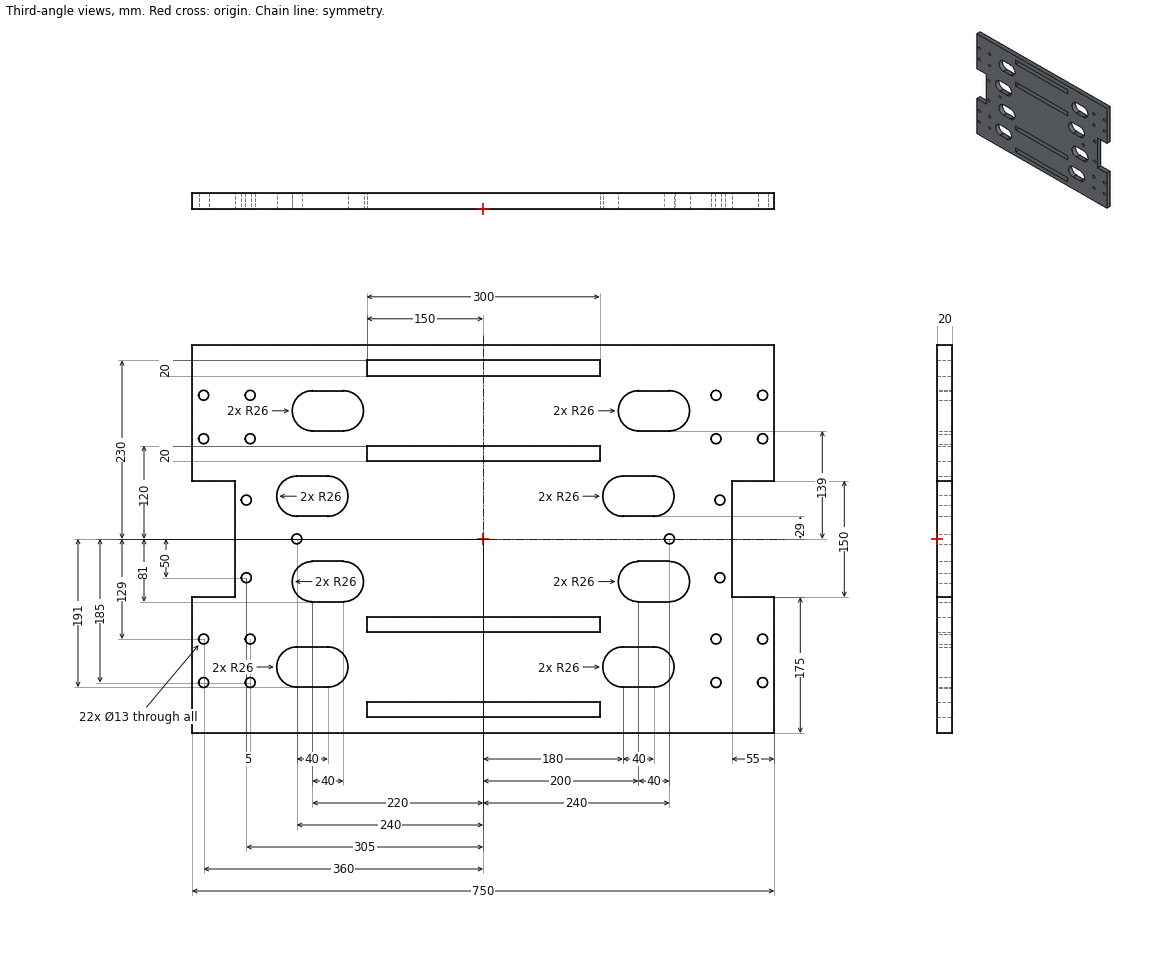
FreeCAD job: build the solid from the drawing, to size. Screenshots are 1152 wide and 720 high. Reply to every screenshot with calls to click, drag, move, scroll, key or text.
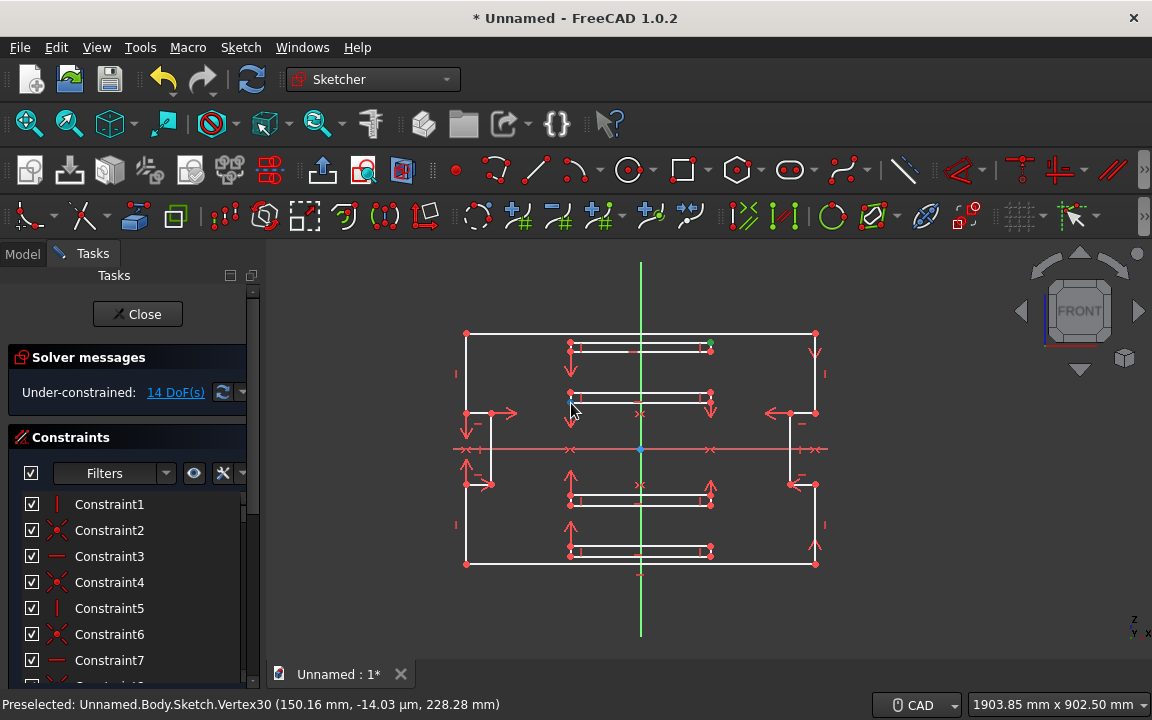
click(711, 557)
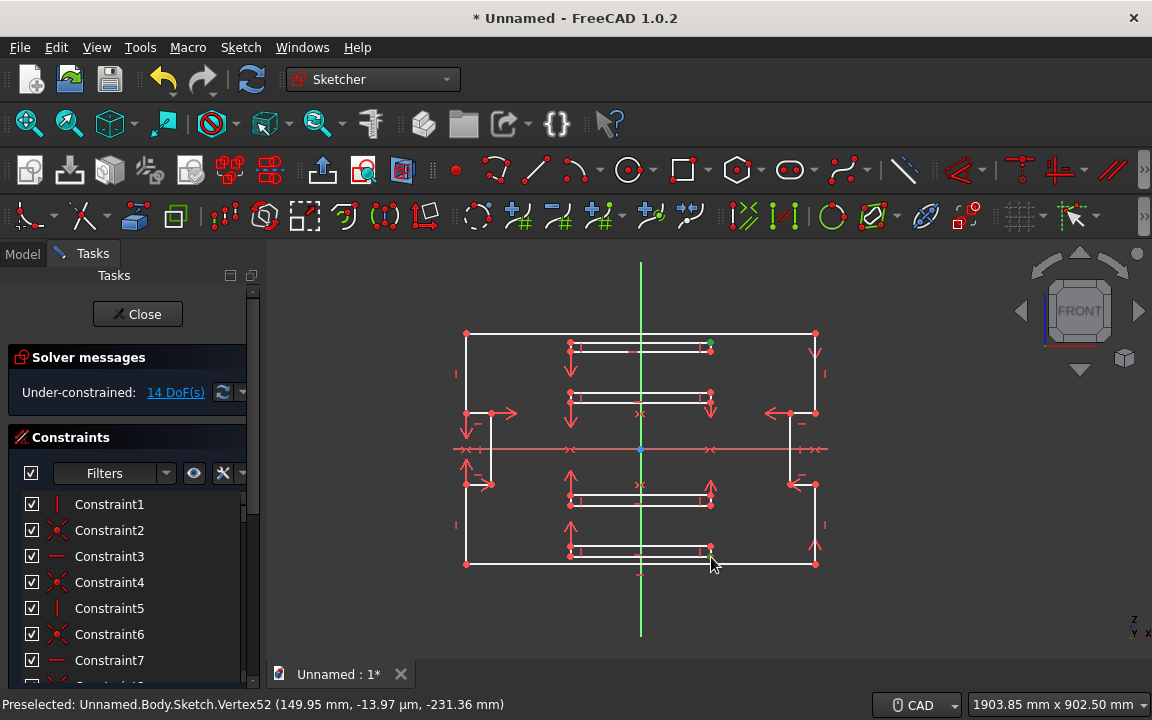
click(542, 449)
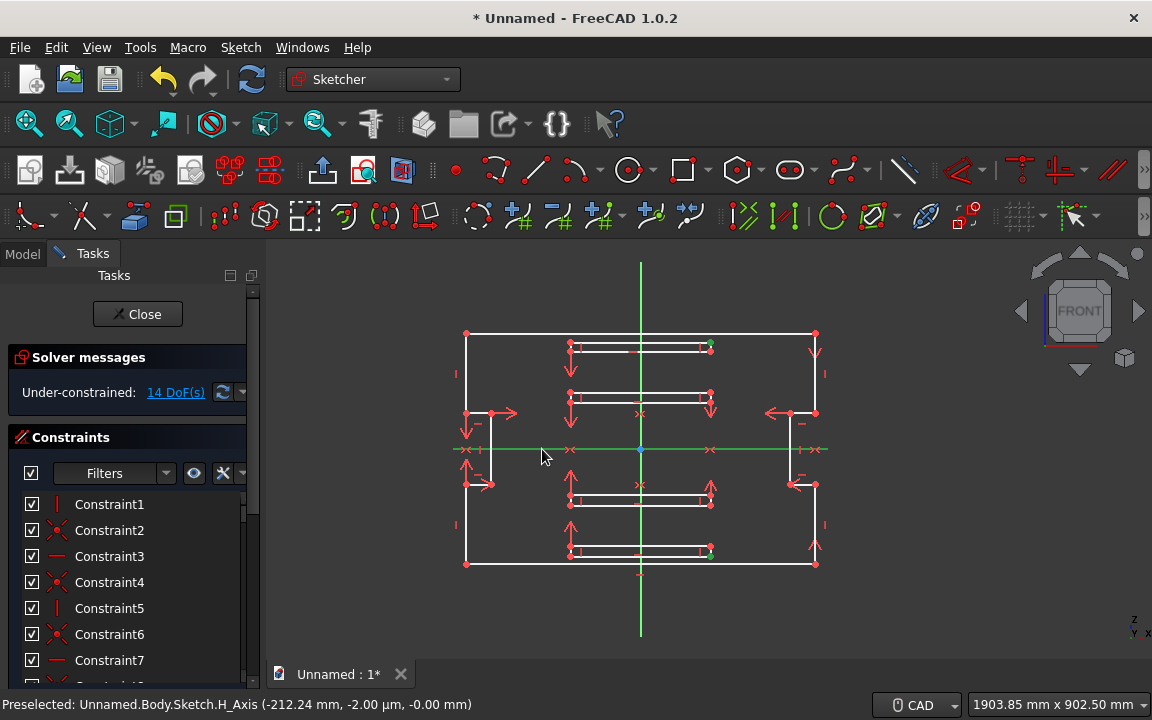
key(s)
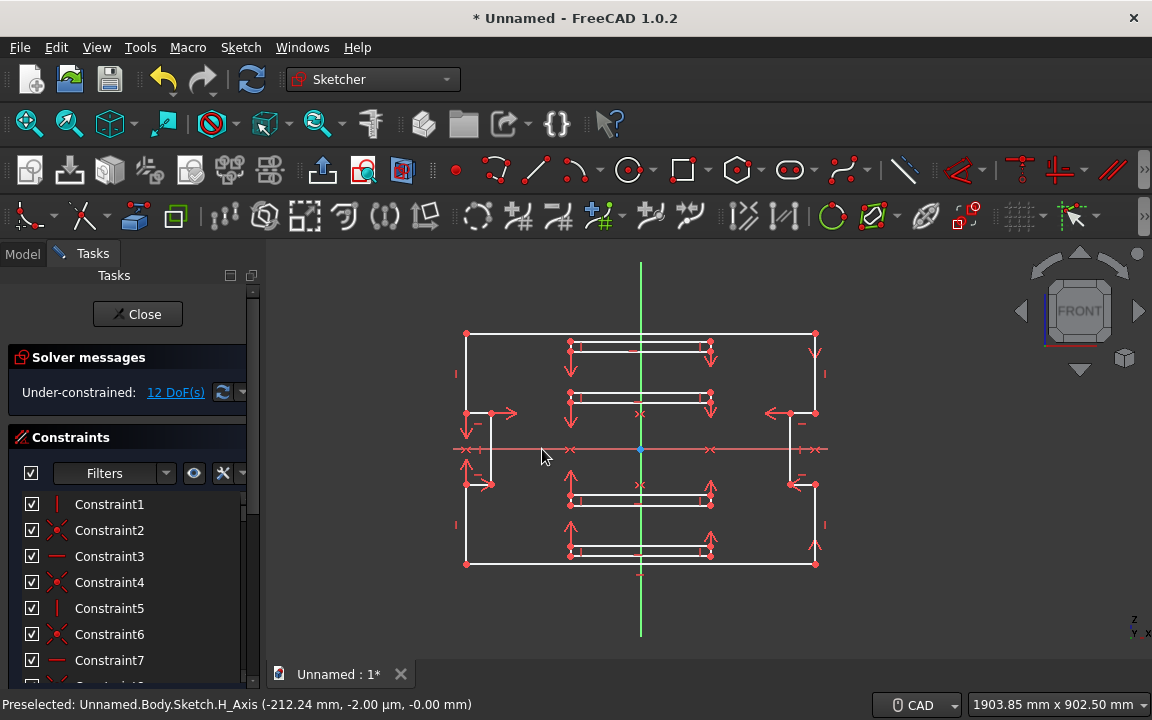
click(958, 170)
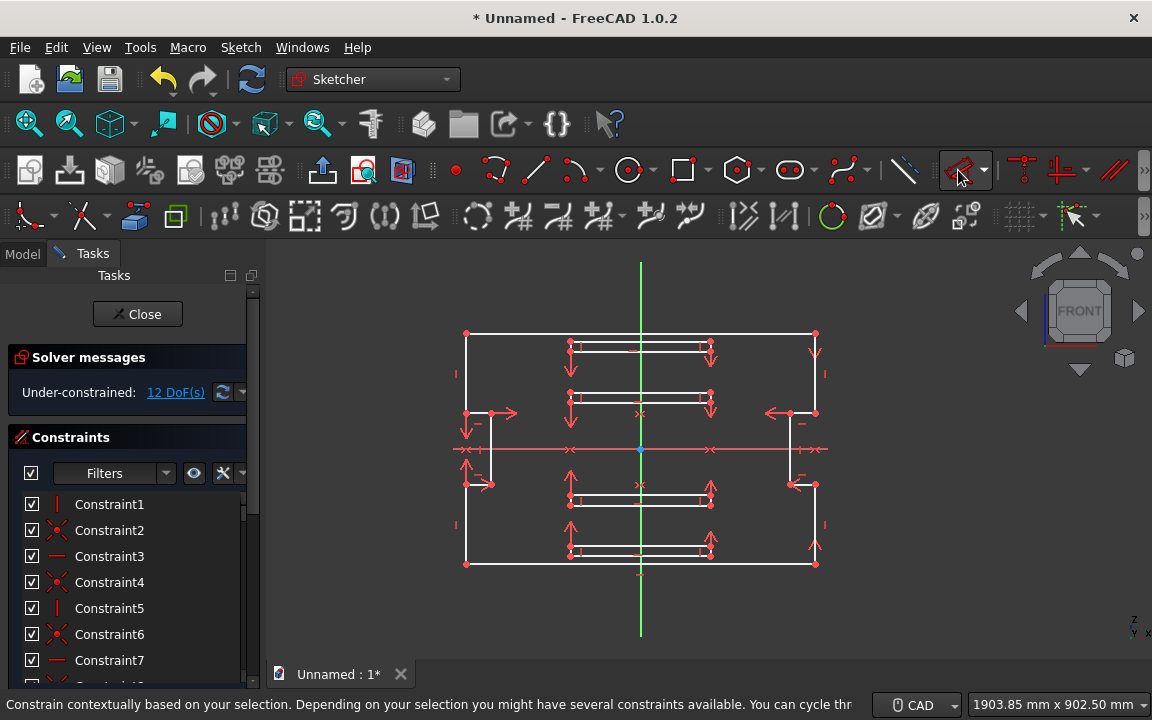
scroll(800, 485, up, 3)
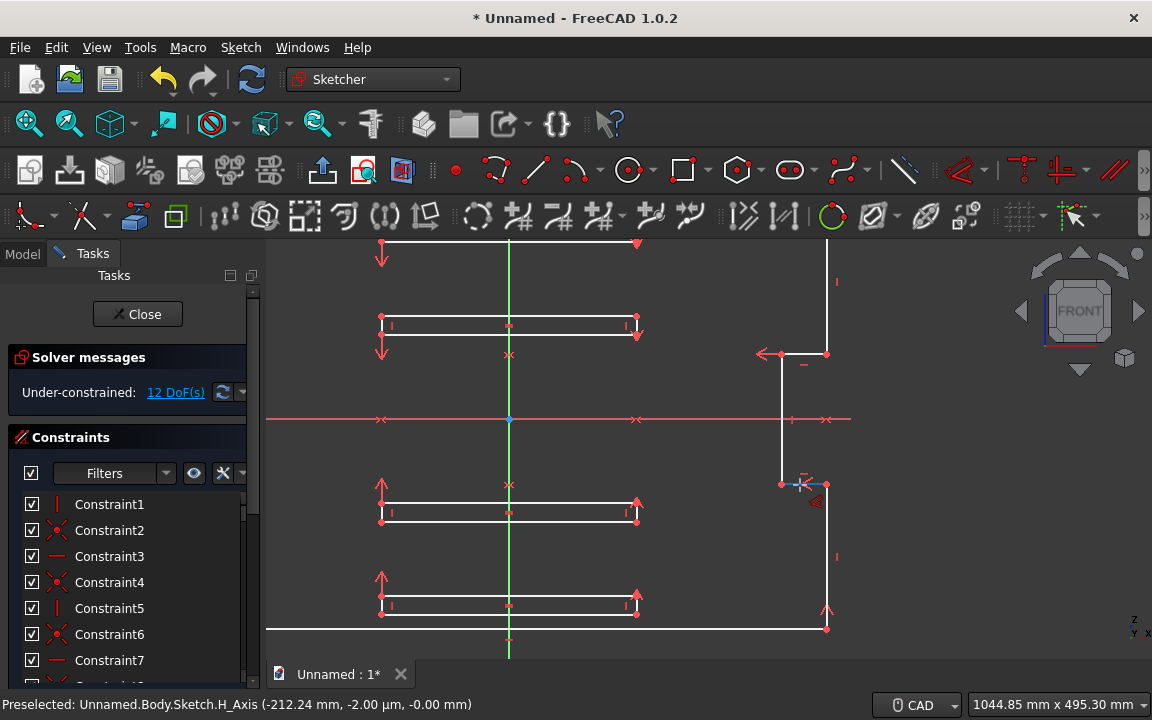
click(800, 484)
click(804, 518)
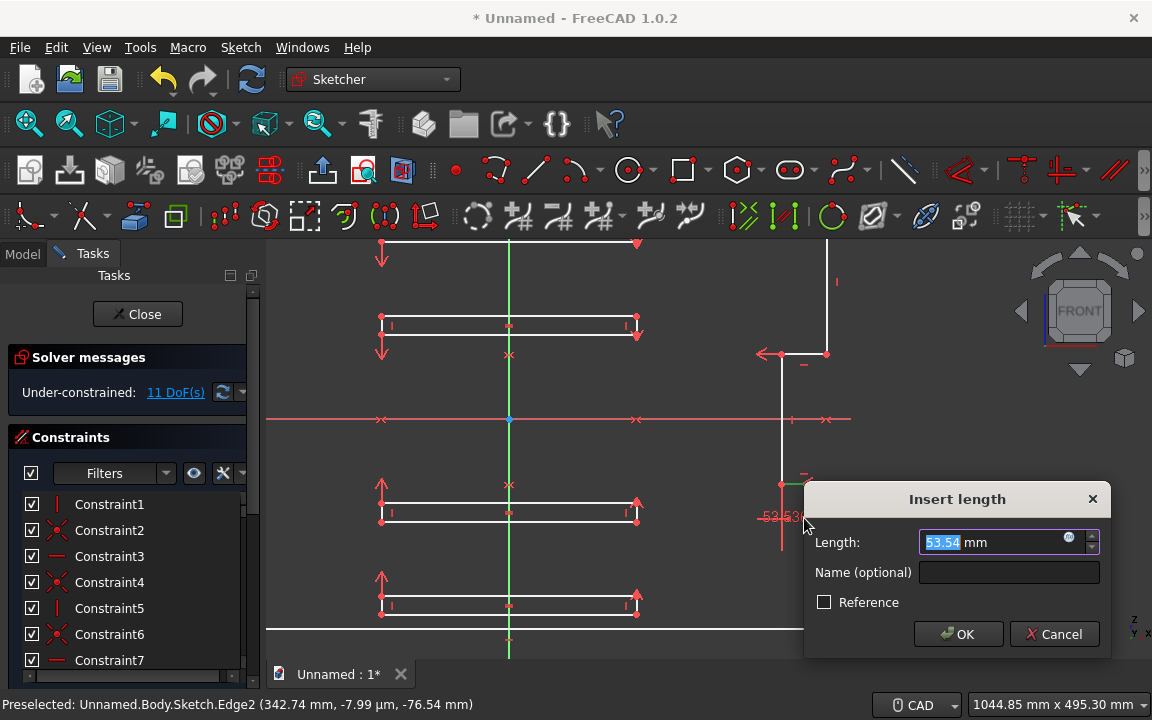
text(55)
key(Return)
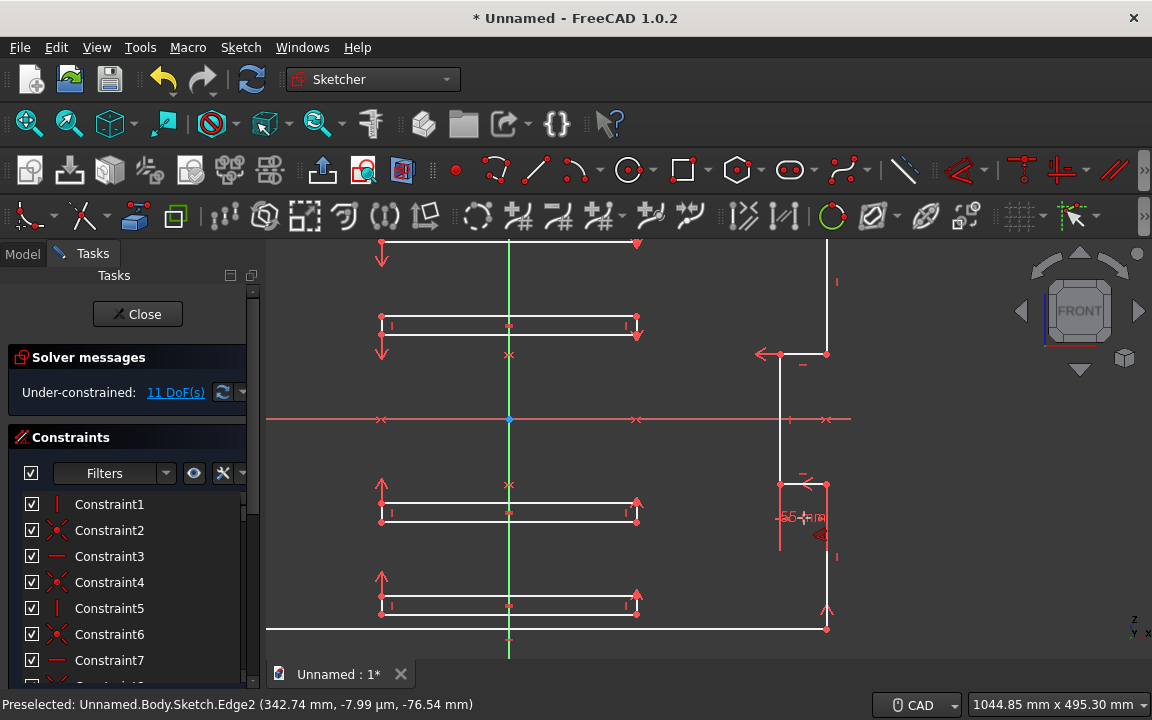
scroll(800, 485, down, 3)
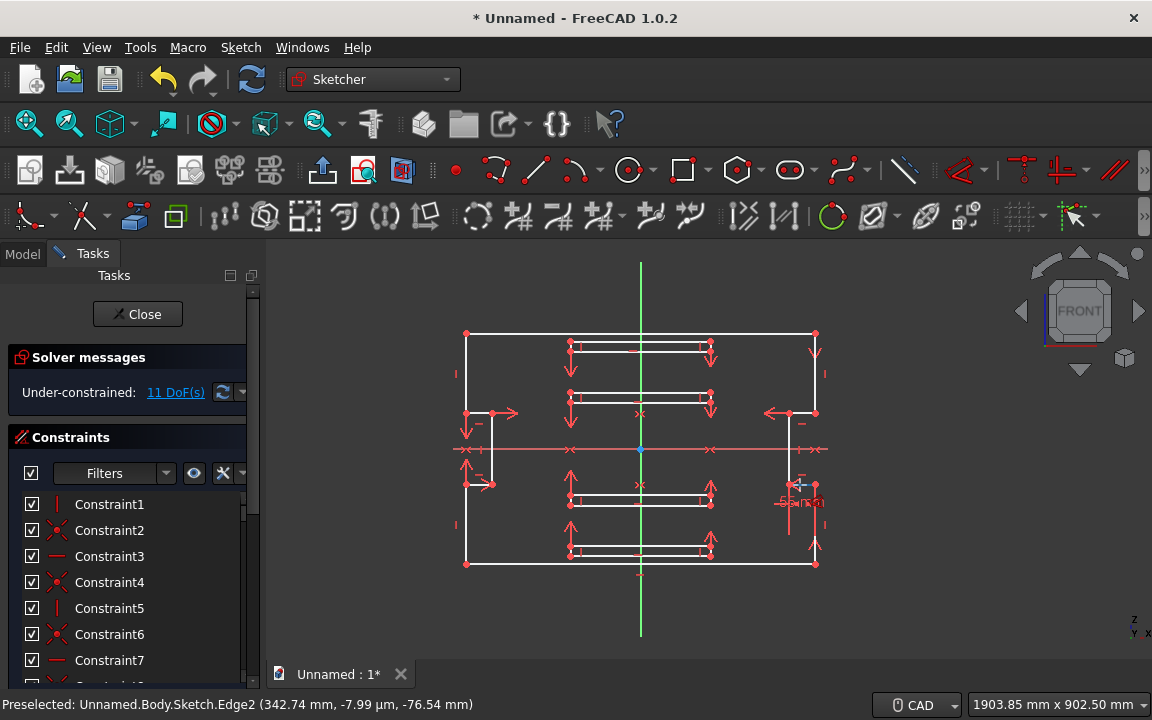
scroll(571, 347, up, 8)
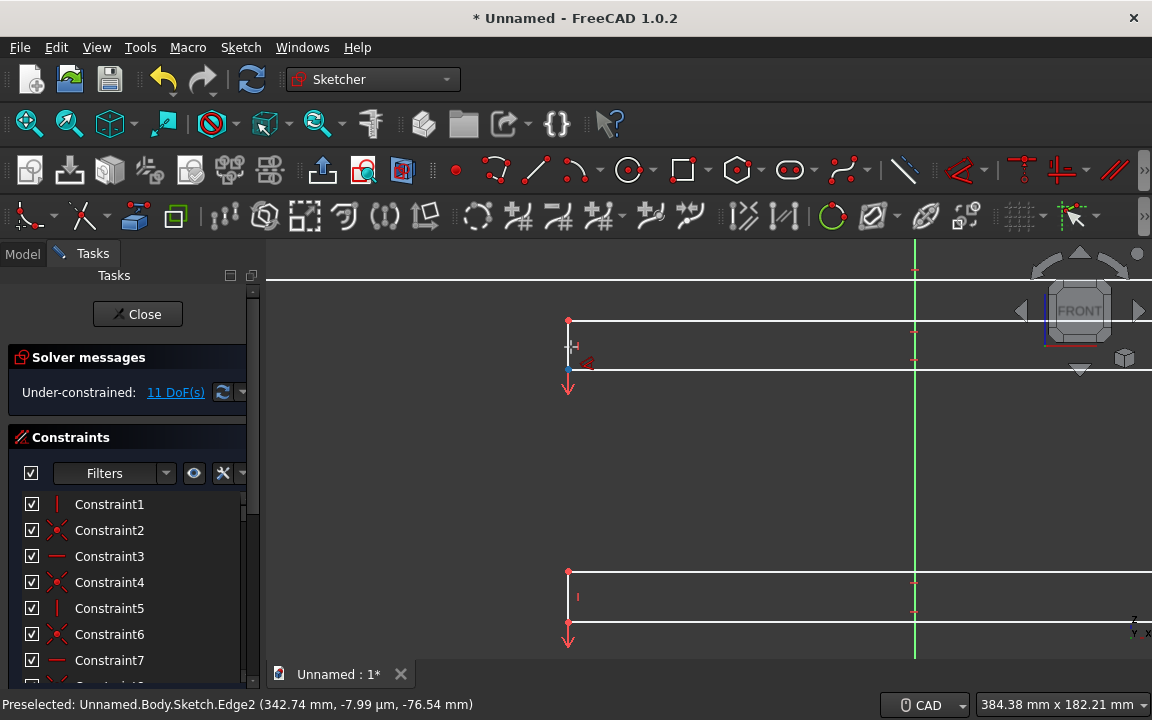
click(568, 345)
click(534, 345)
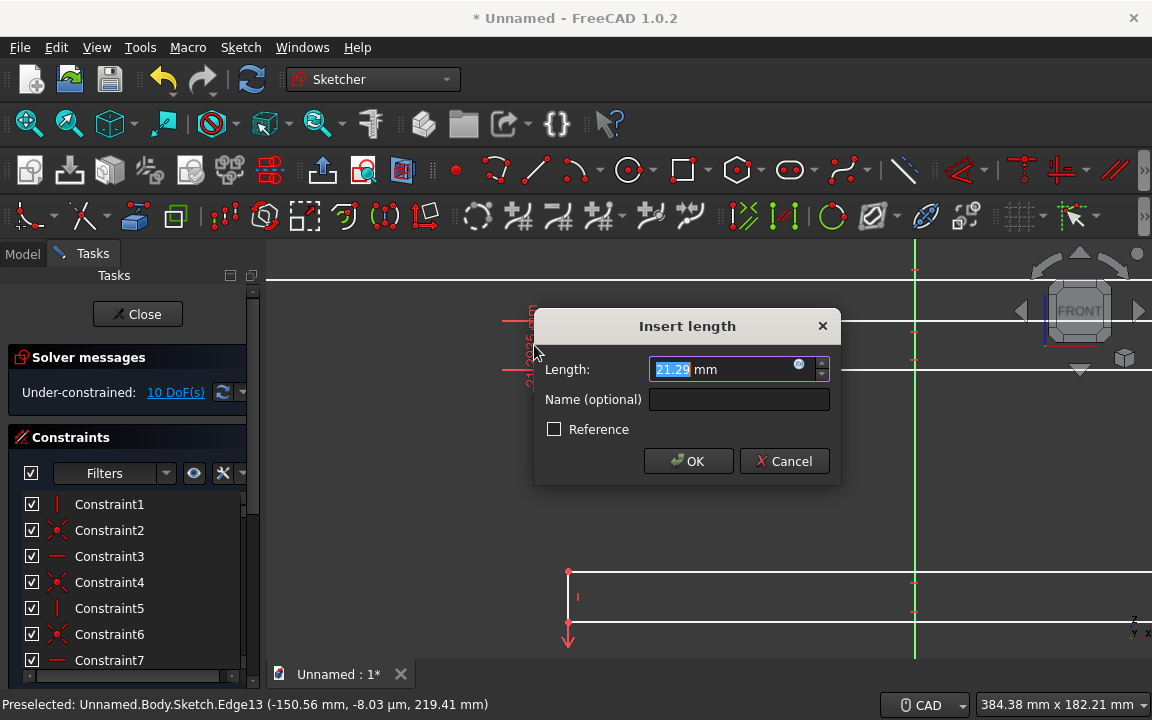
text(20)
key(Return)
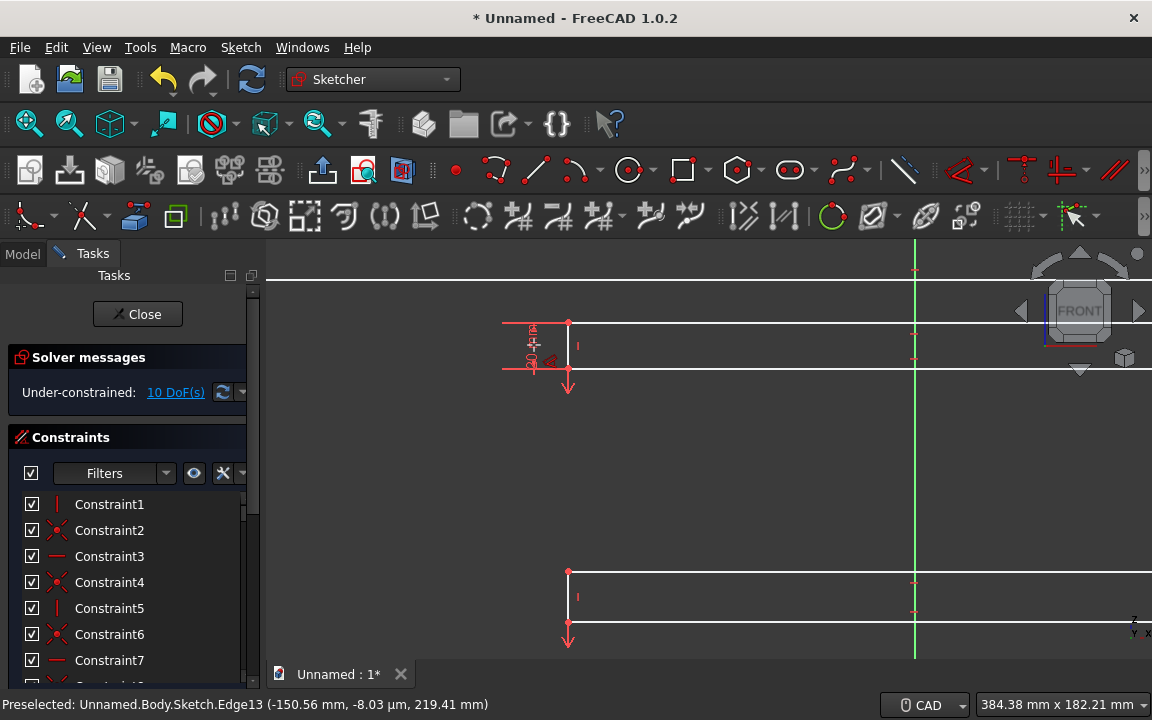
click(568, 587)
click(534, 597)